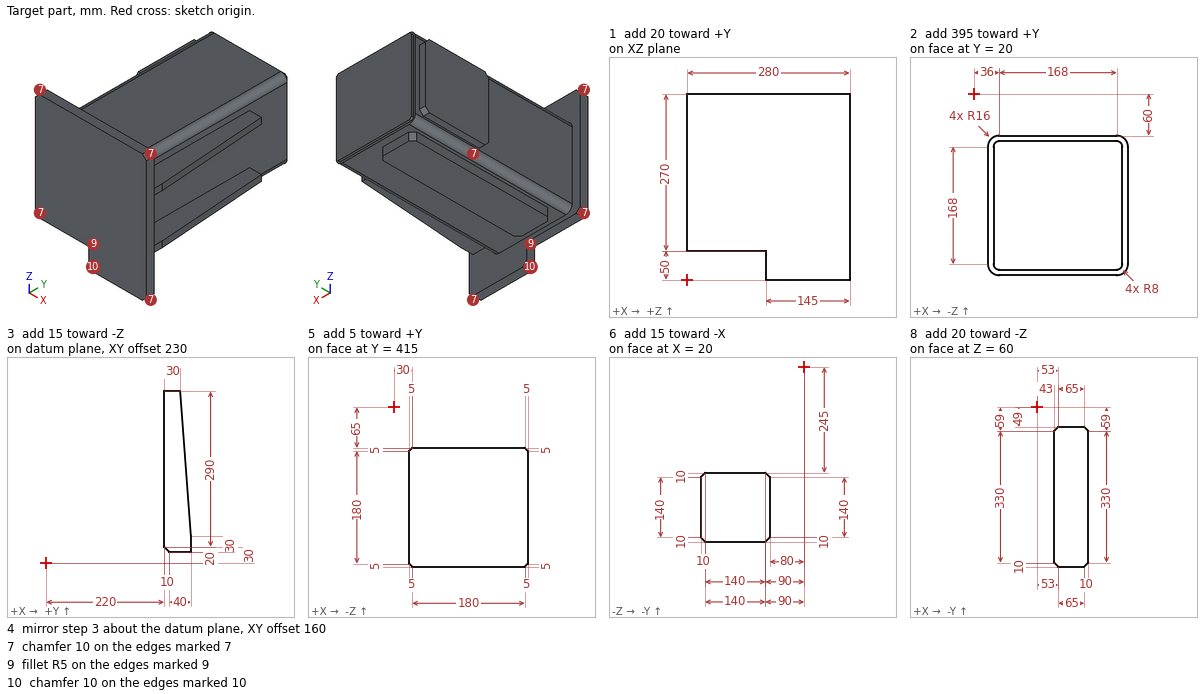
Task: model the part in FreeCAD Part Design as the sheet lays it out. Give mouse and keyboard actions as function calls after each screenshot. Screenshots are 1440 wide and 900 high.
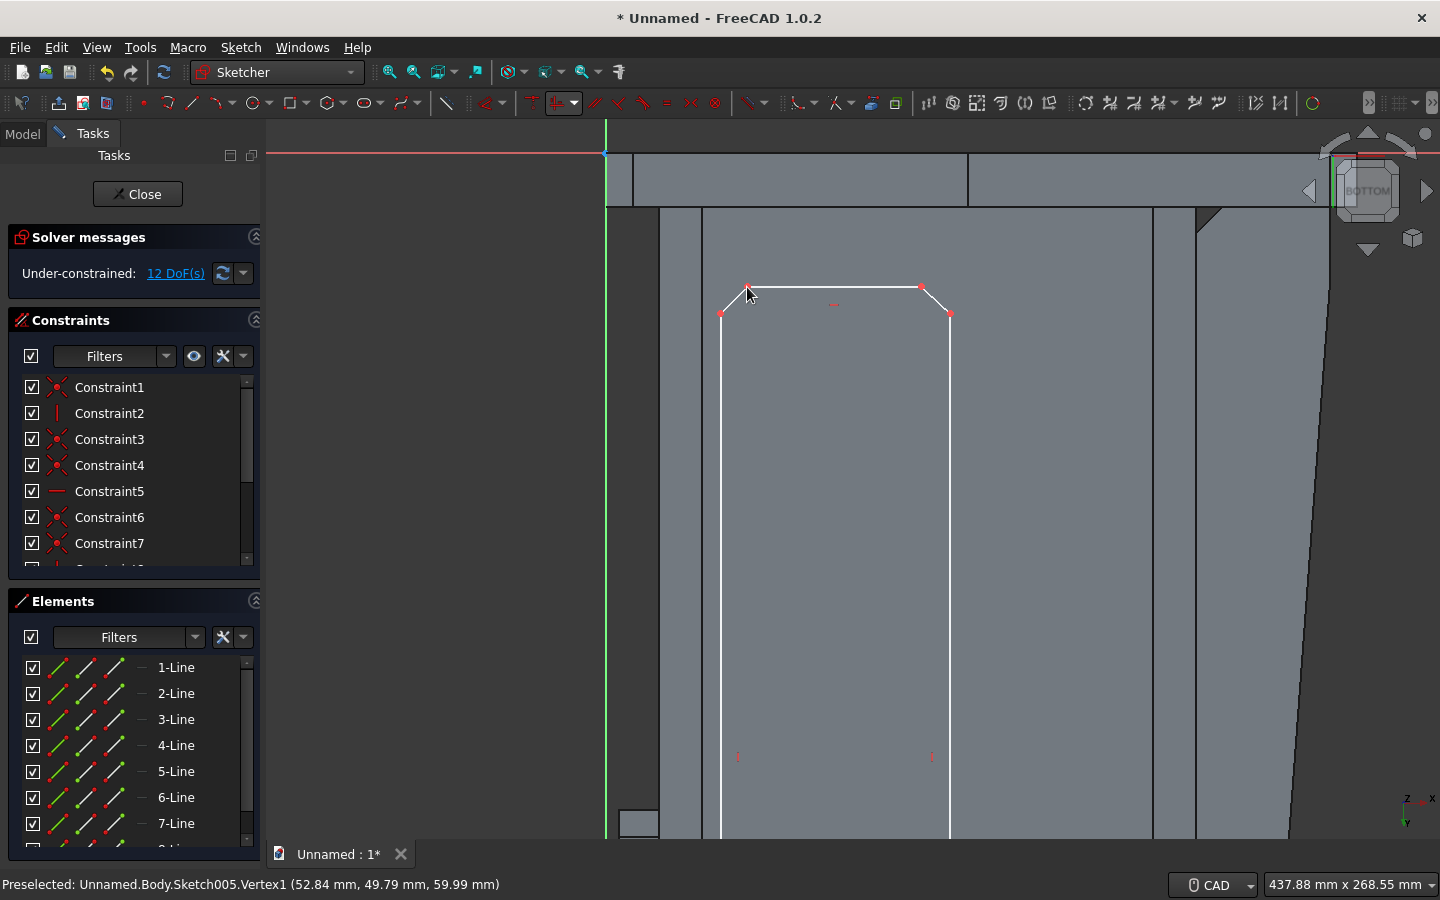
click(486, 104)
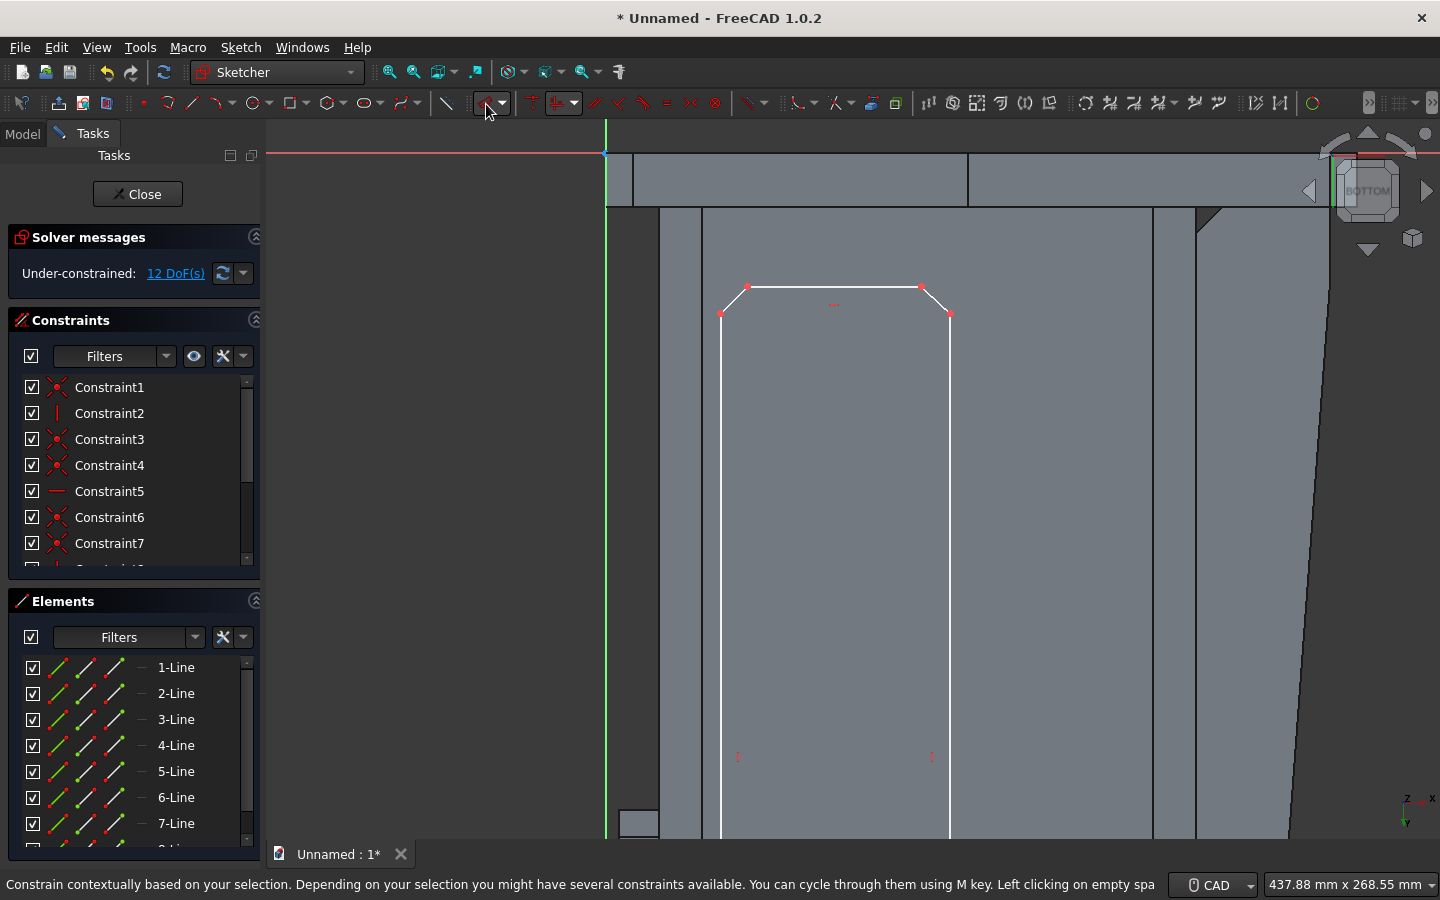
scroll(790, 308, down, 4)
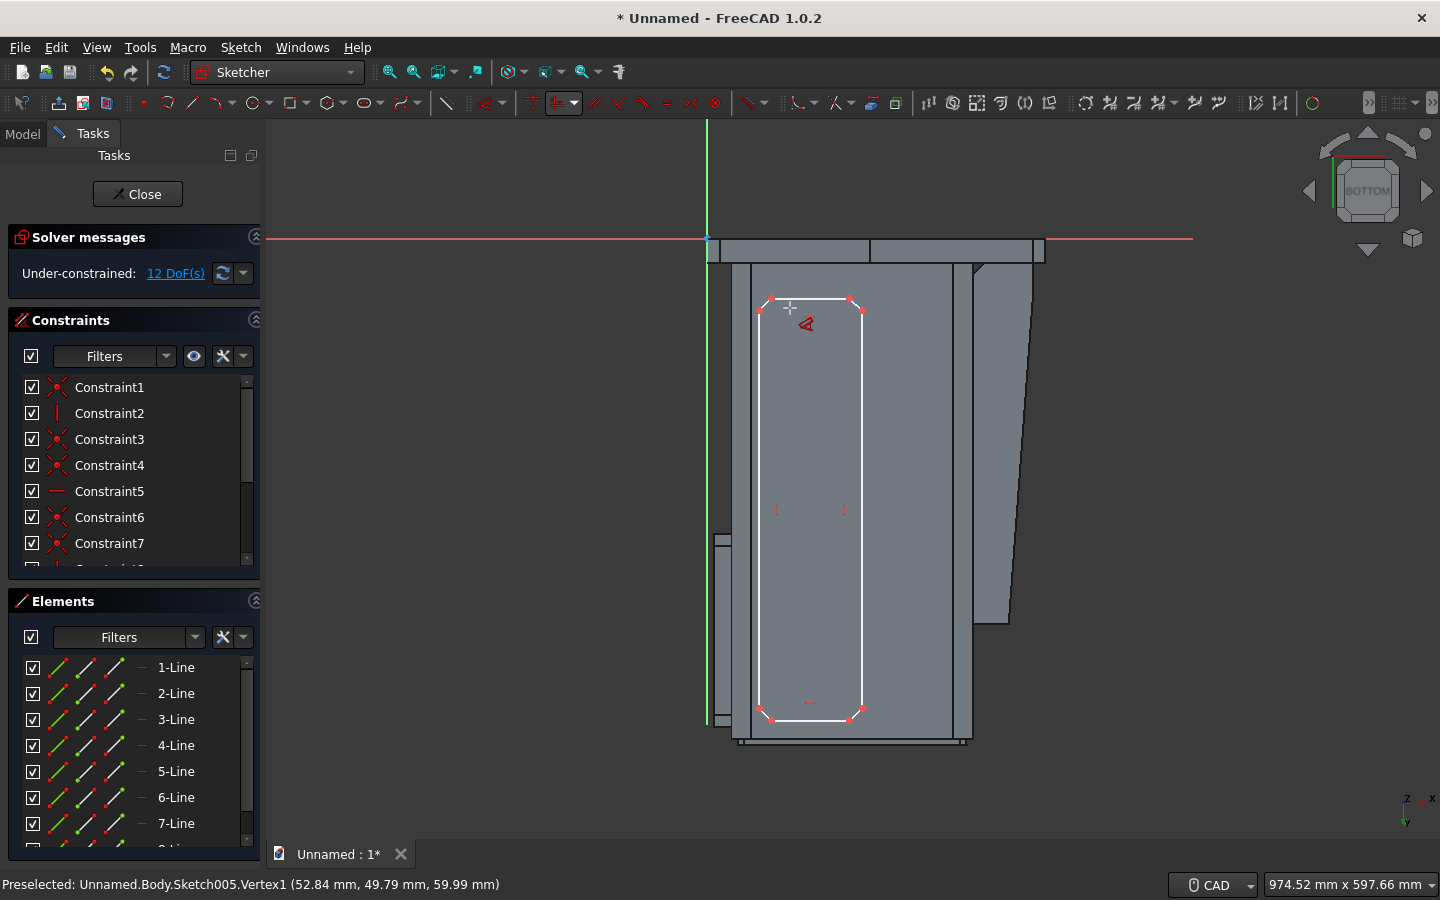
click(795, 721)
click(810, 755)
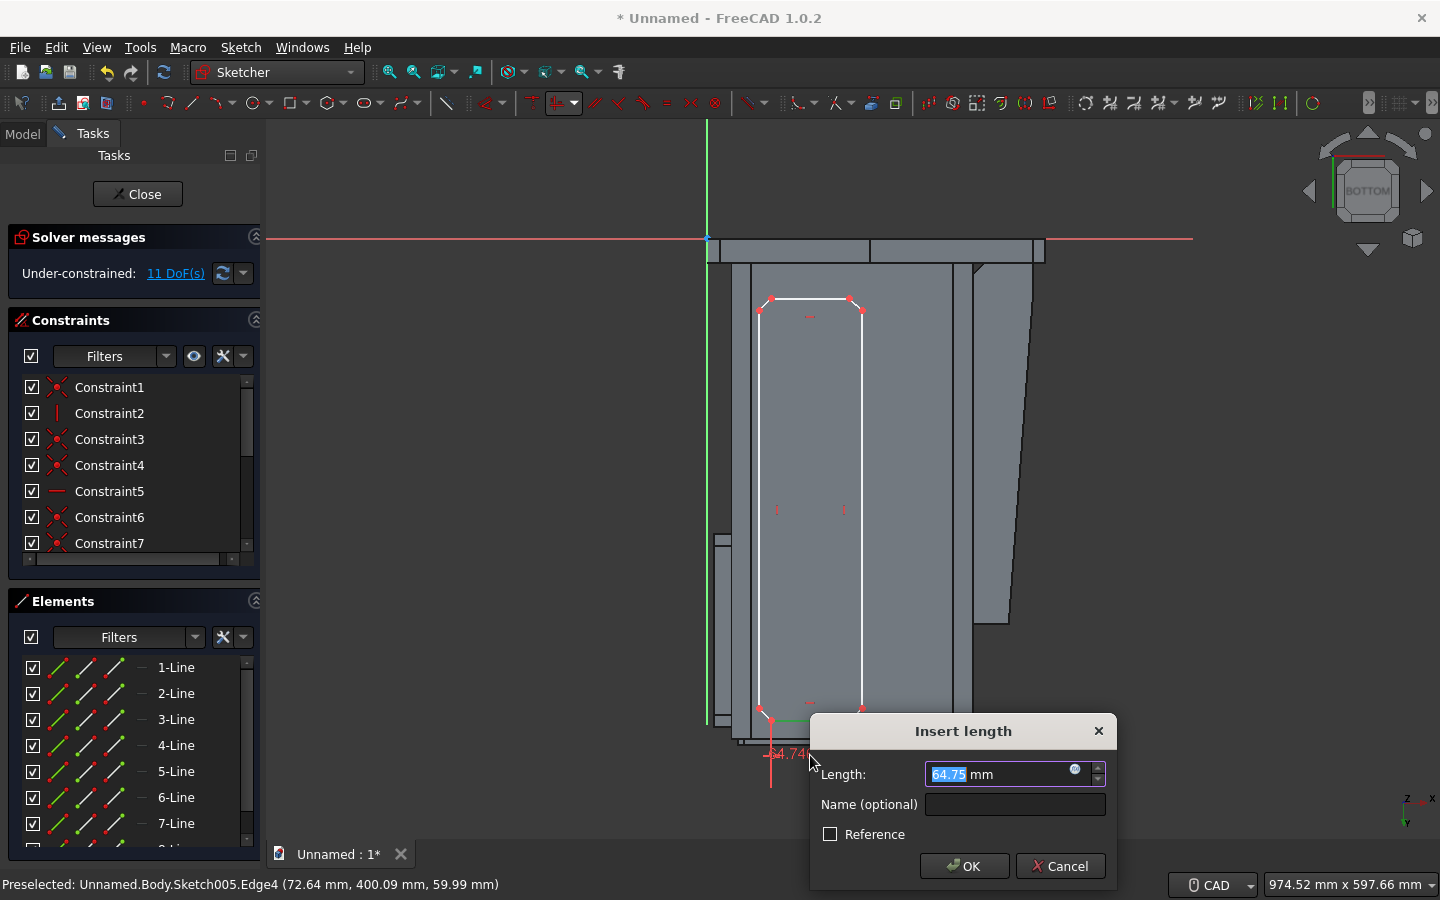
text(65)
key(Return)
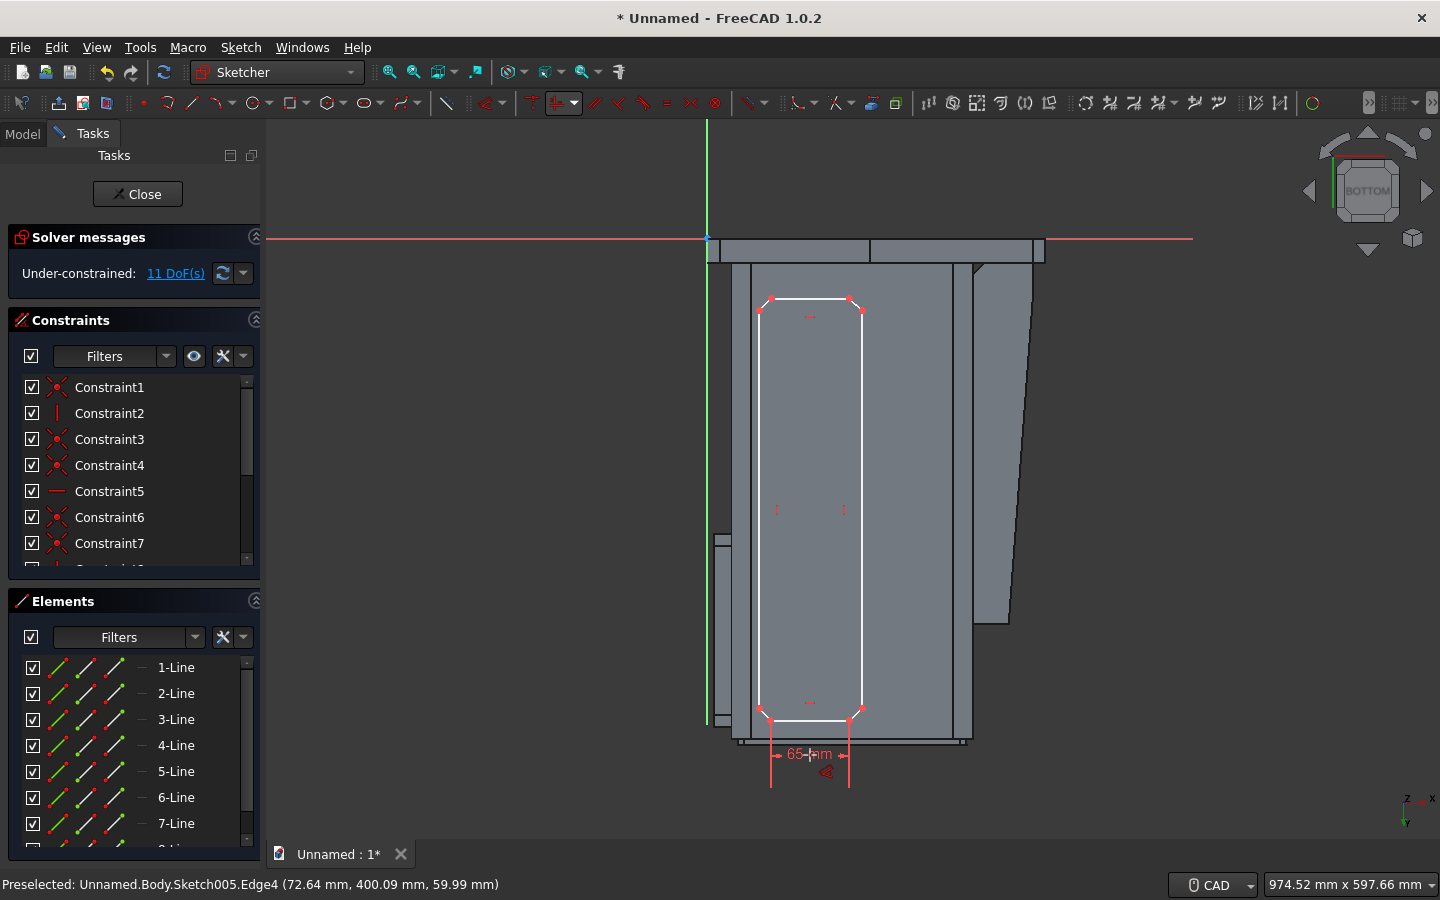
click(826, 299)
click(810, 265)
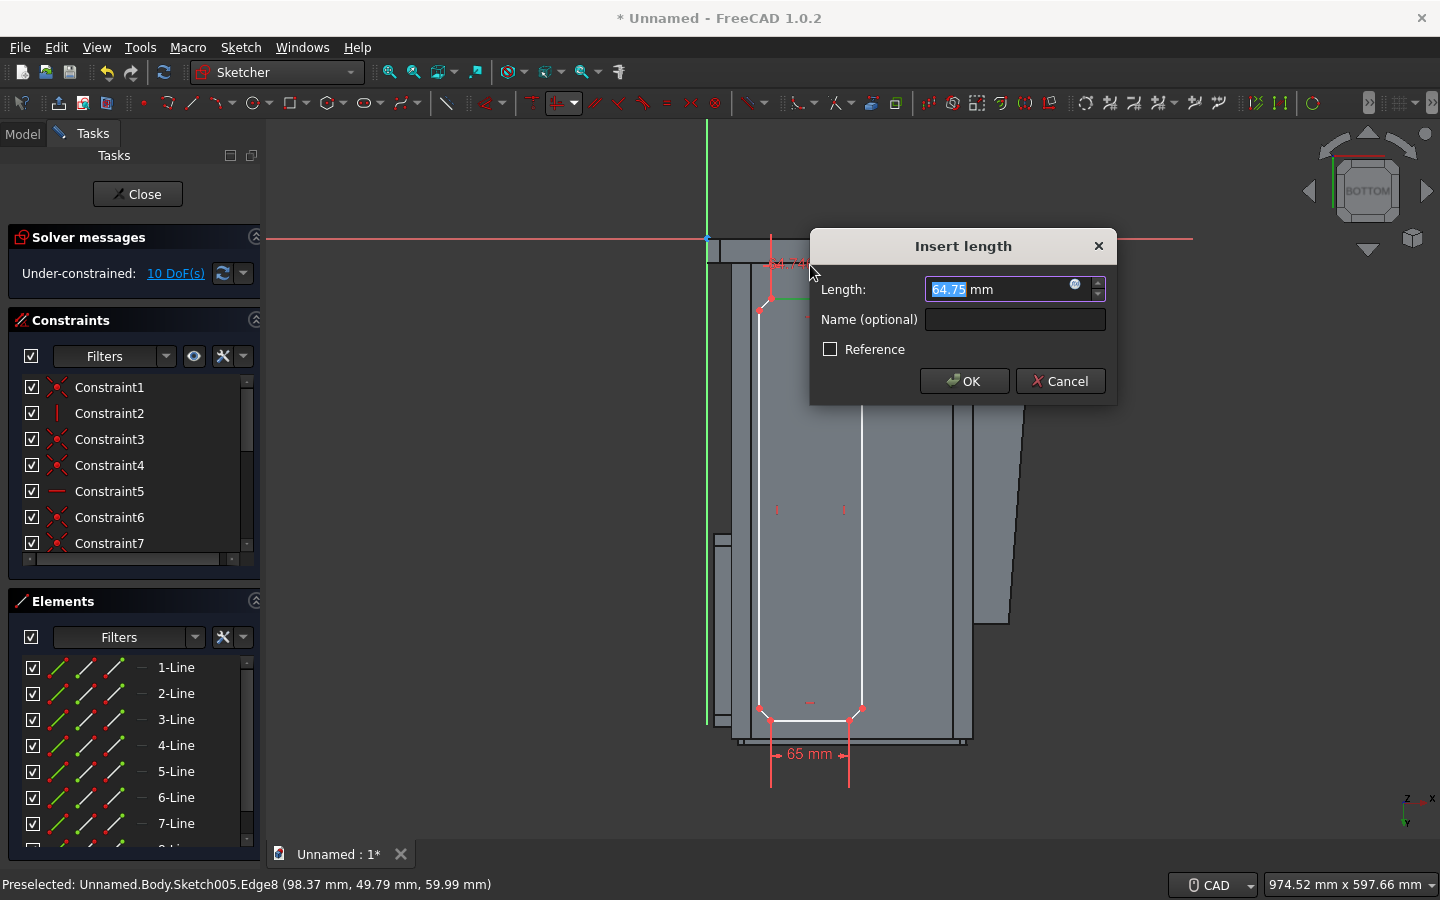
text(65)
key(Return)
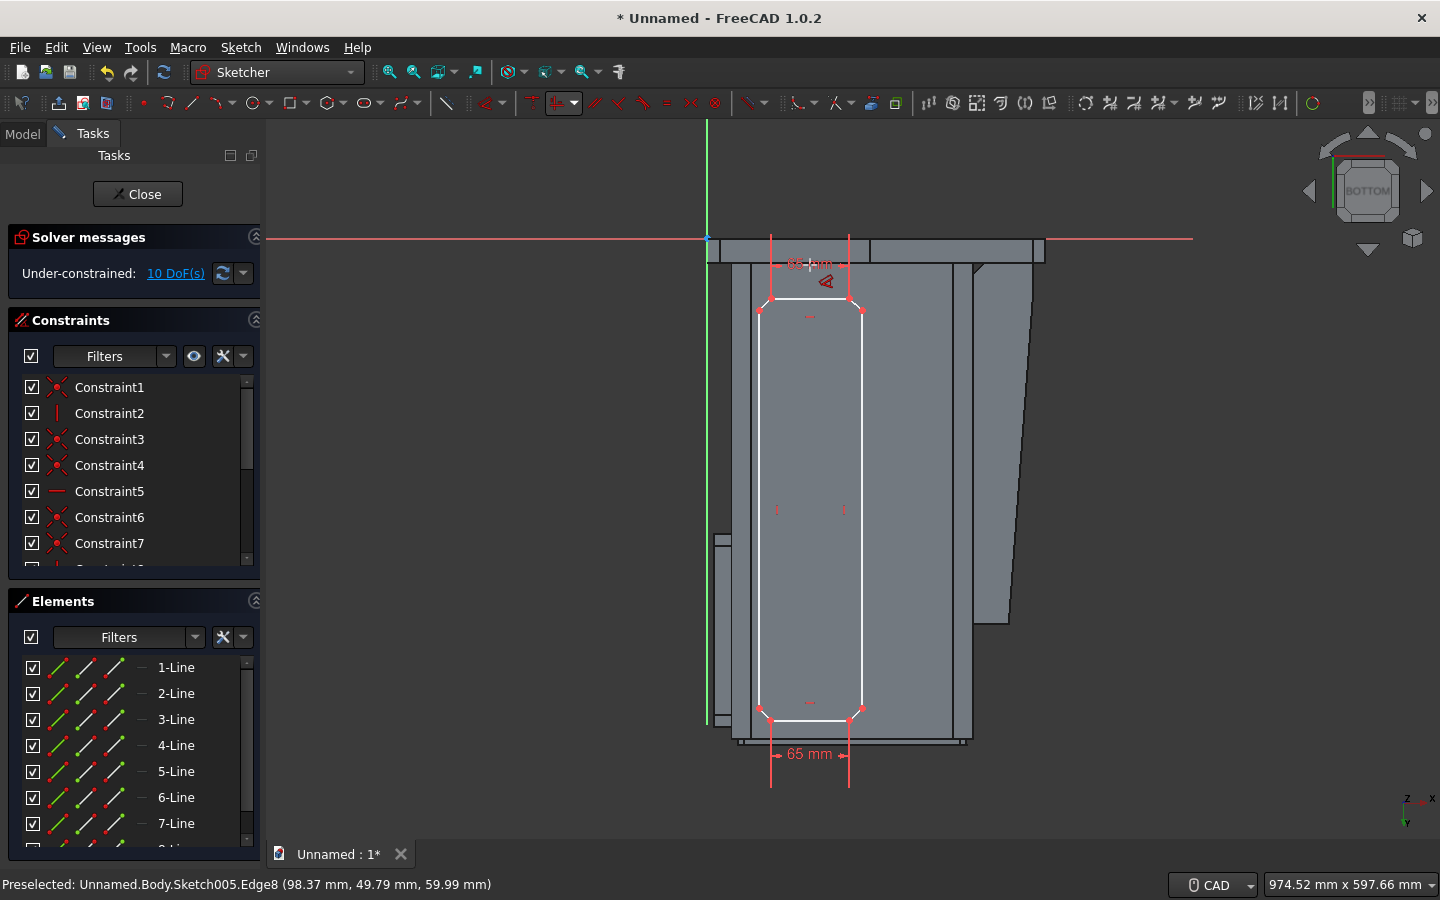
click(759, 430)
click(725, 510)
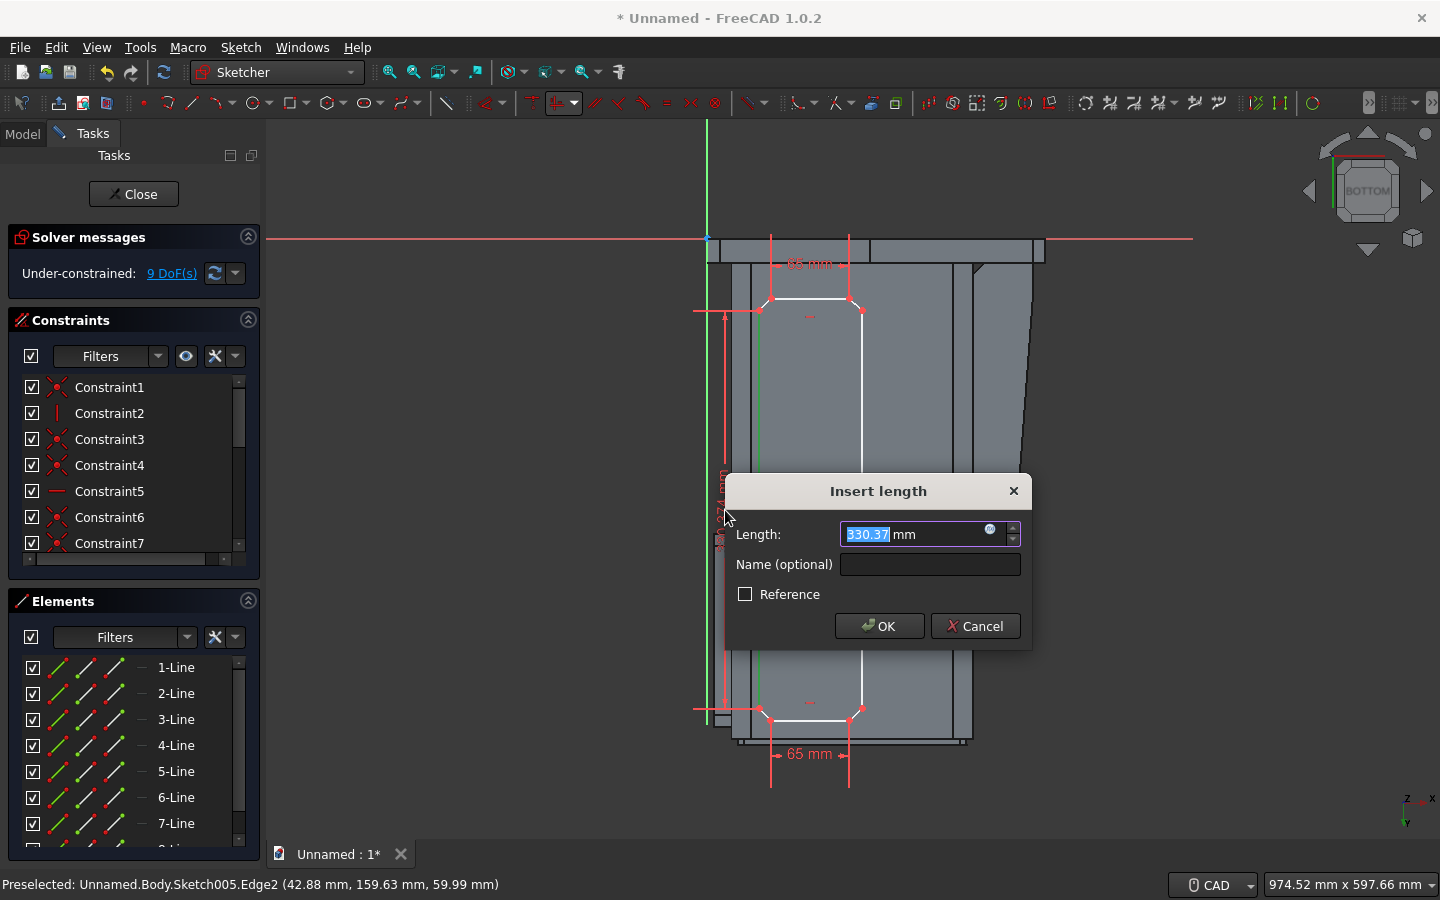
text(330)
key(Return)